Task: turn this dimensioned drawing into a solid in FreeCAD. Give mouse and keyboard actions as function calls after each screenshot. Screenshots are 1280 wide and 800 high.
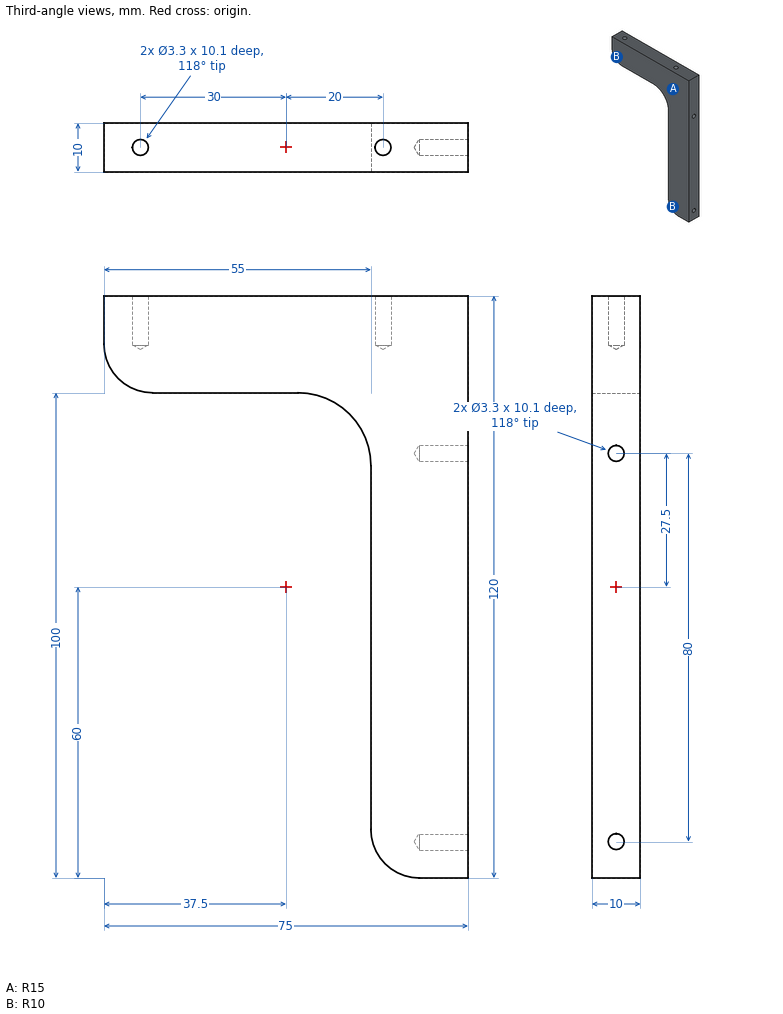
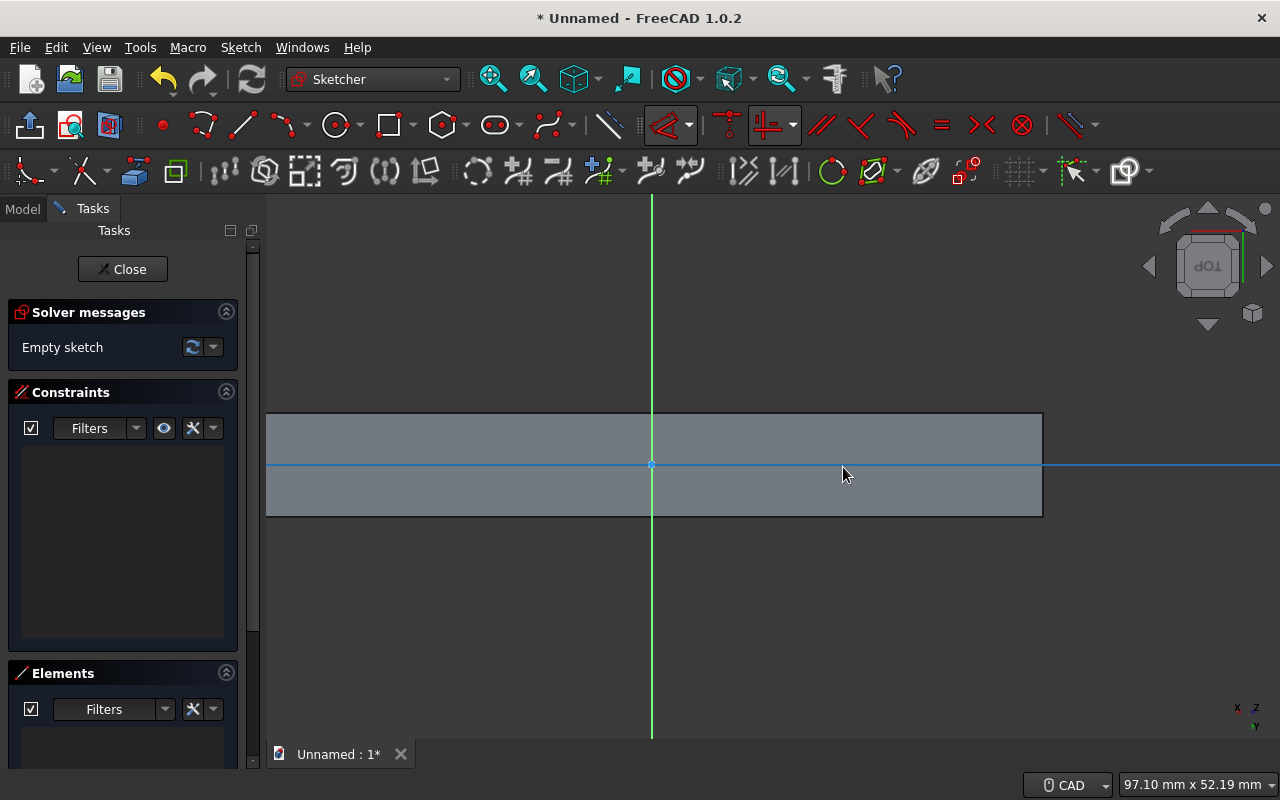
click(336, 126)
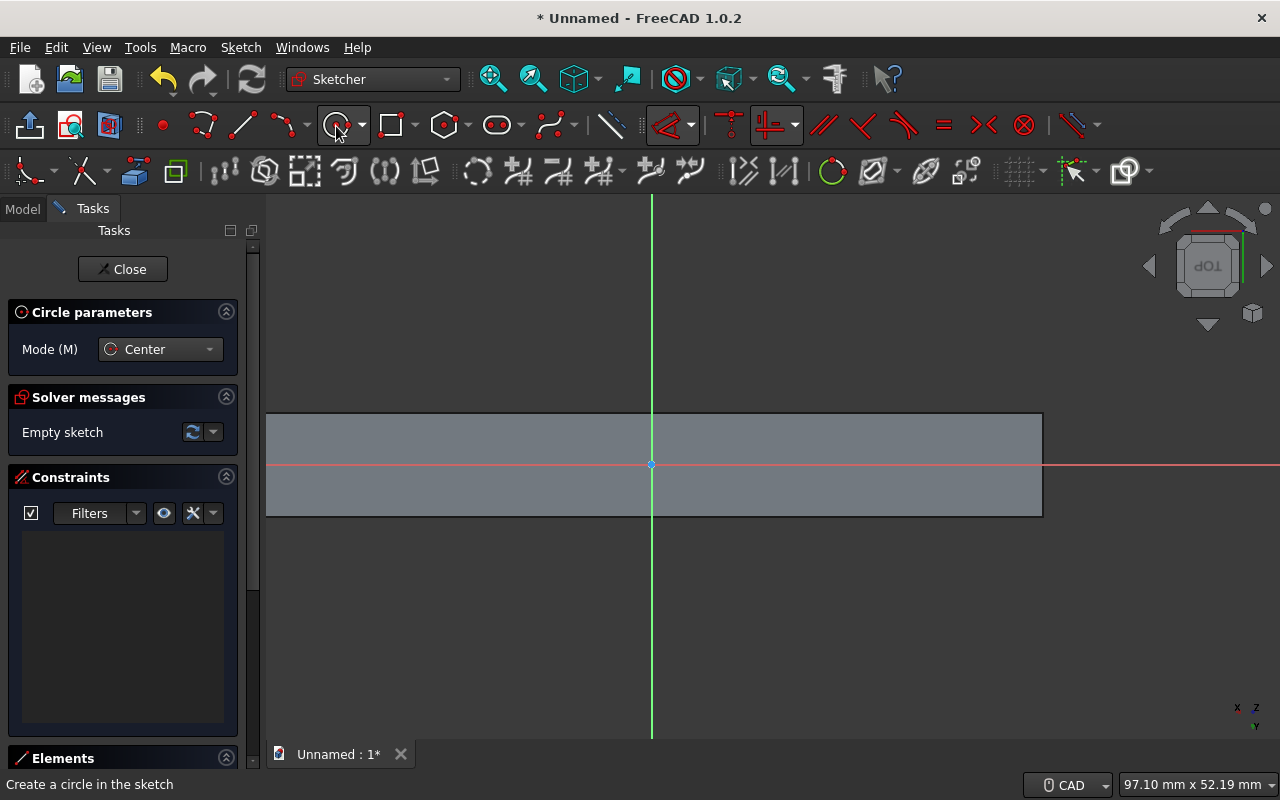
scroll(965, 465, up, 2)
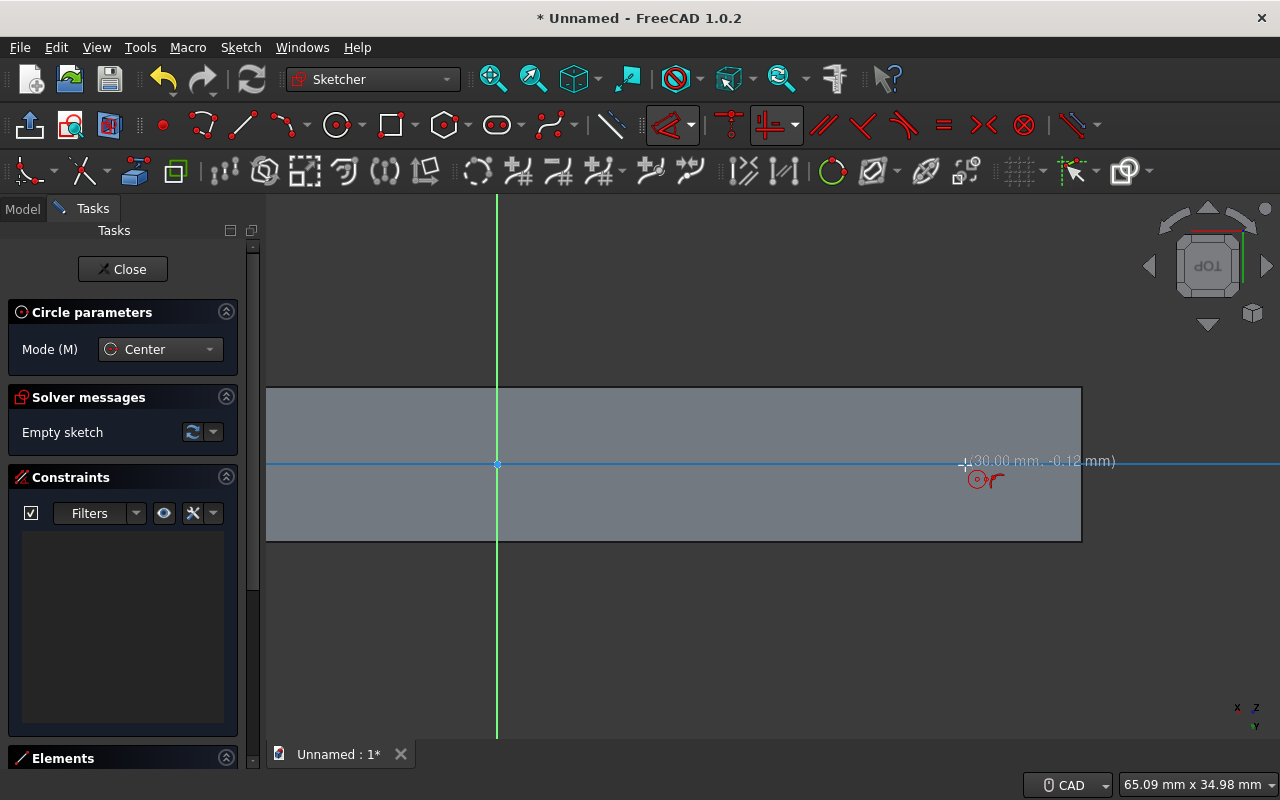
click(965, 464)
click(983, 446)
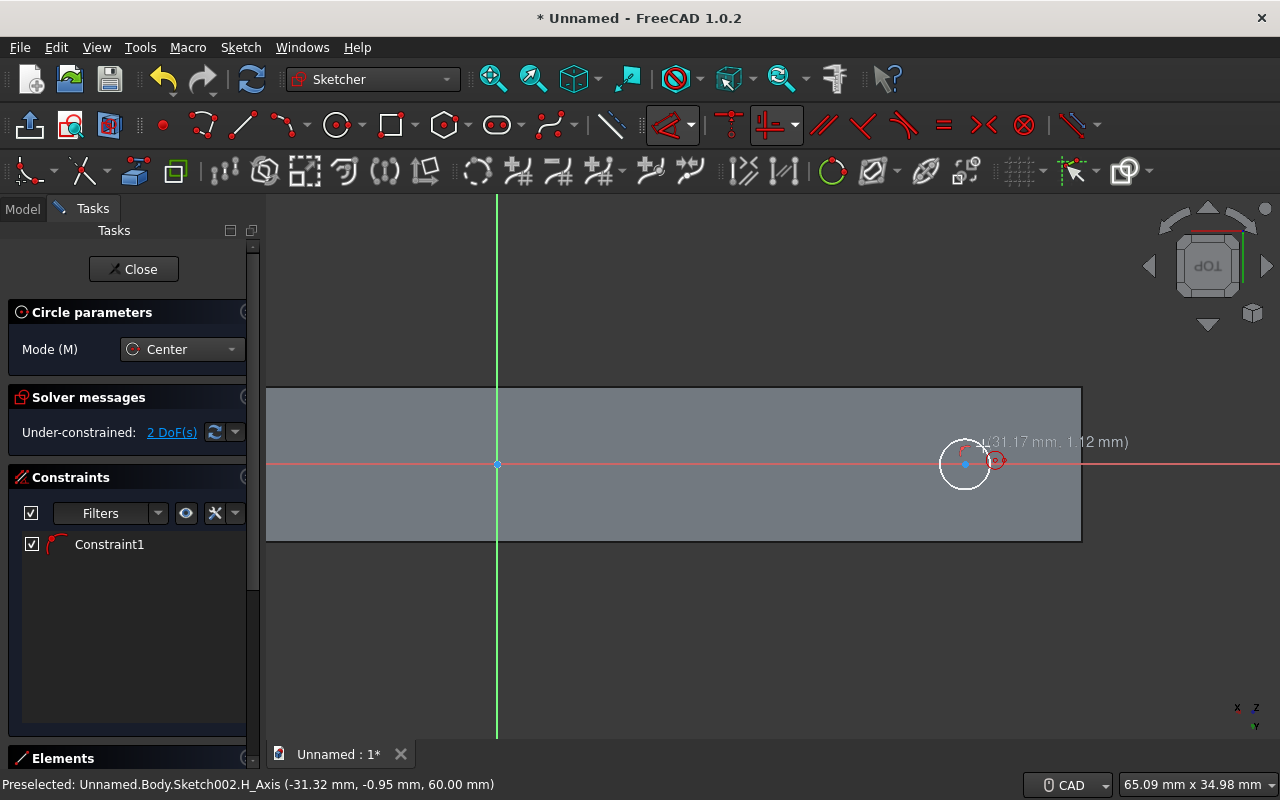
scroll(967, 471, down, 2)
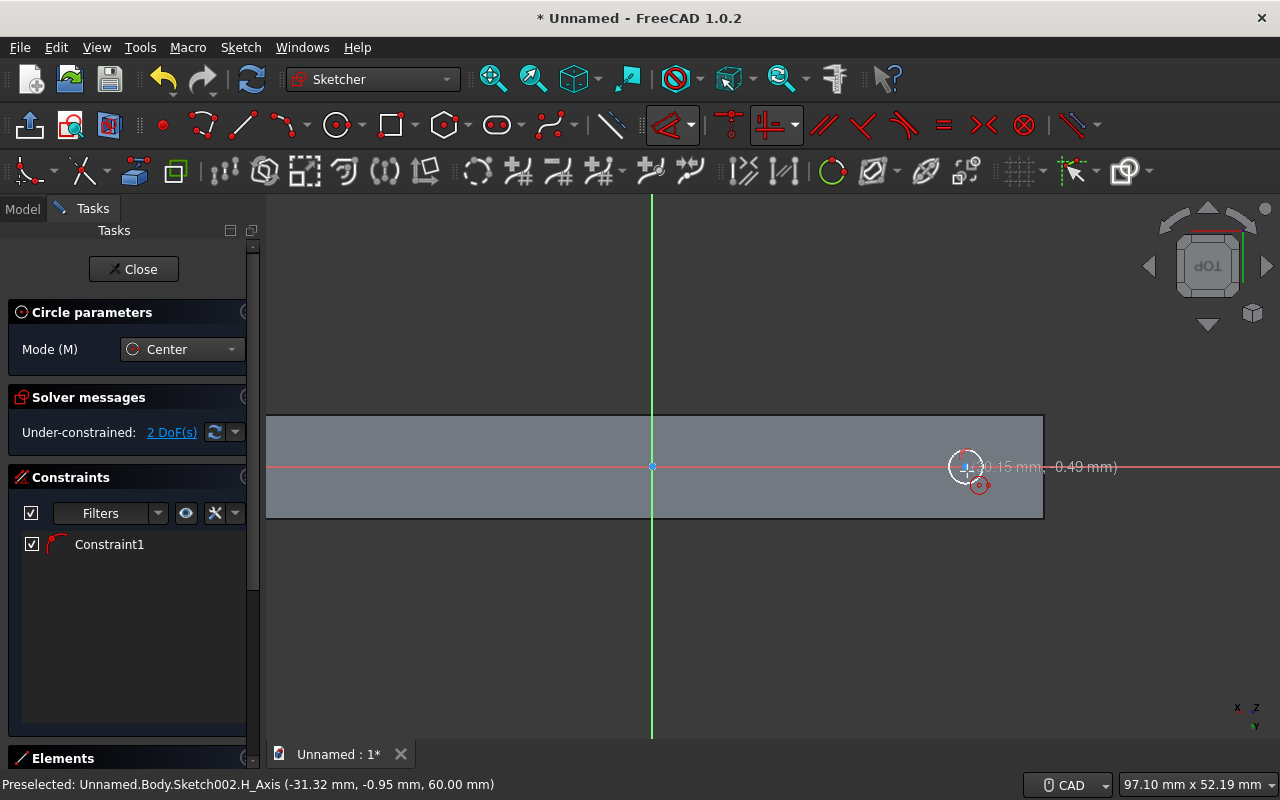
scroll(444, 467, up, 2)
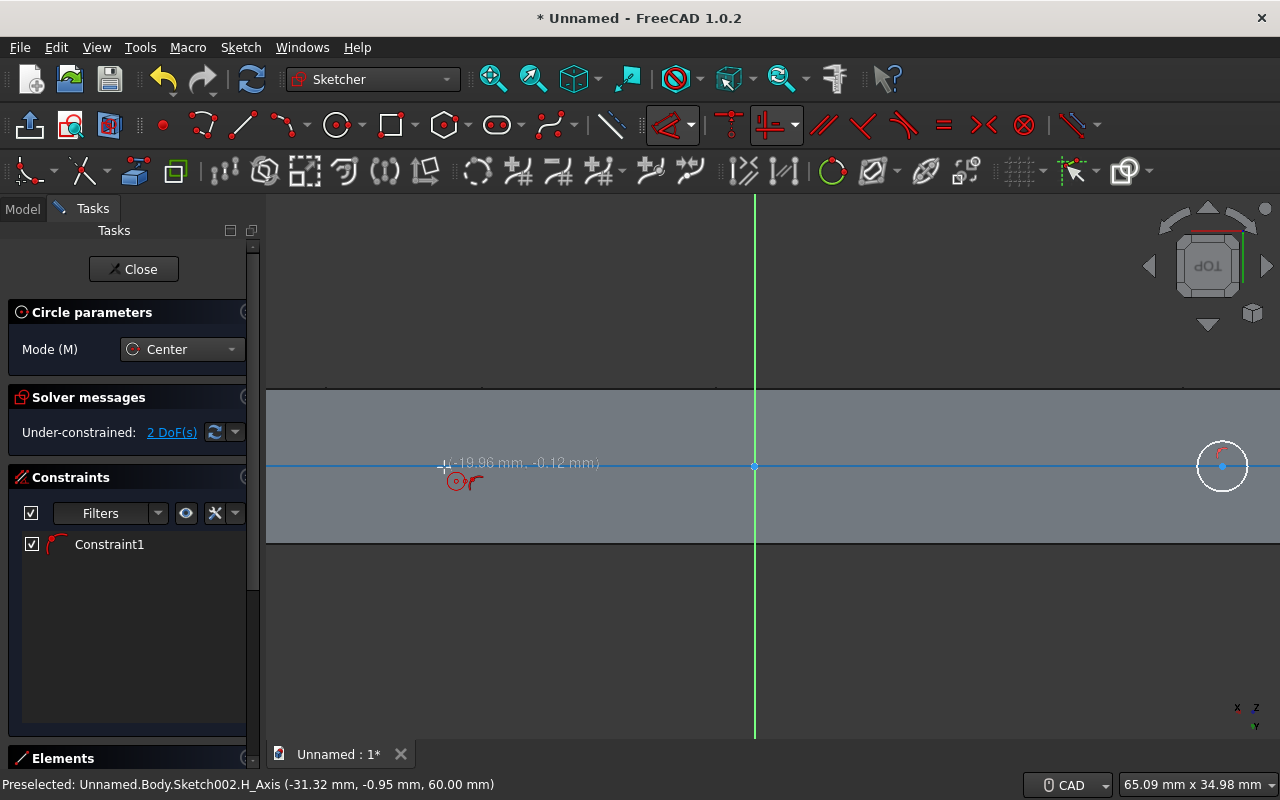
click(443, 466)
click(461, 448)
key(Escape)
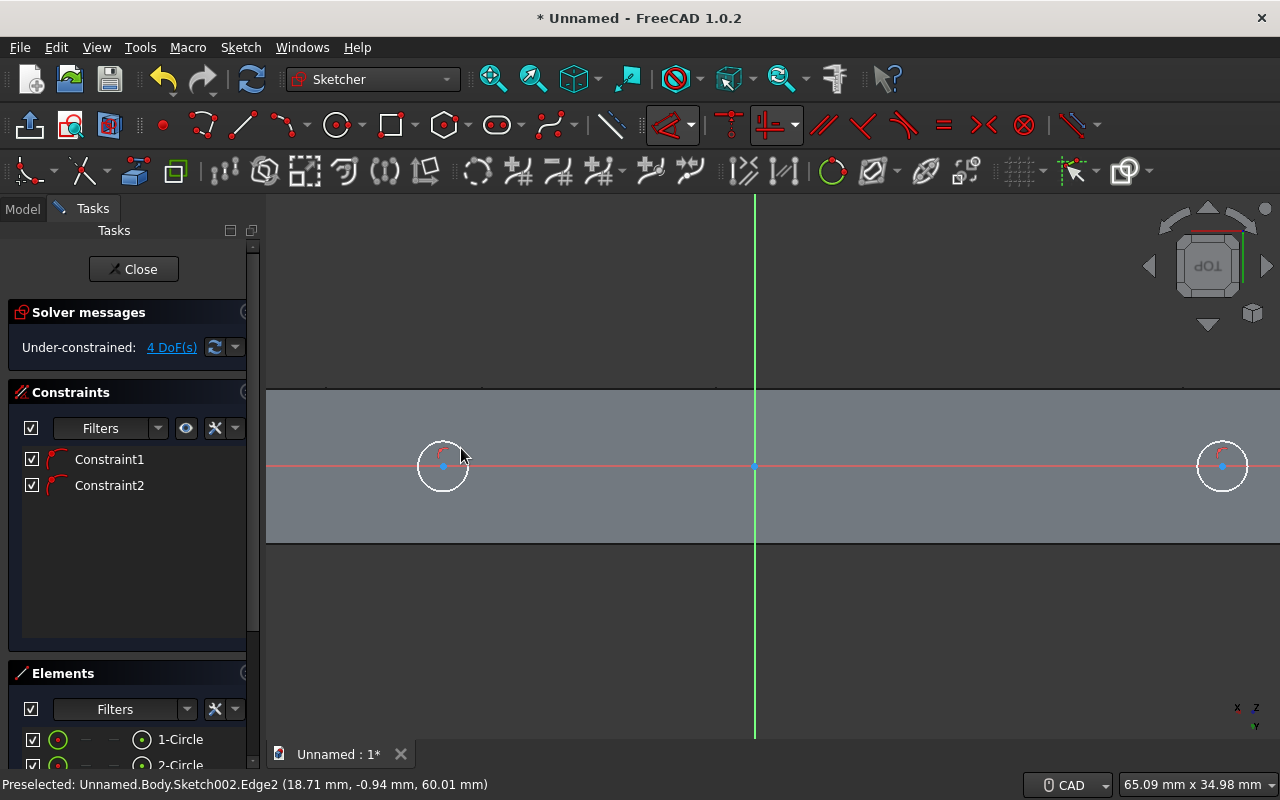
scroll(444, 467, down, 2)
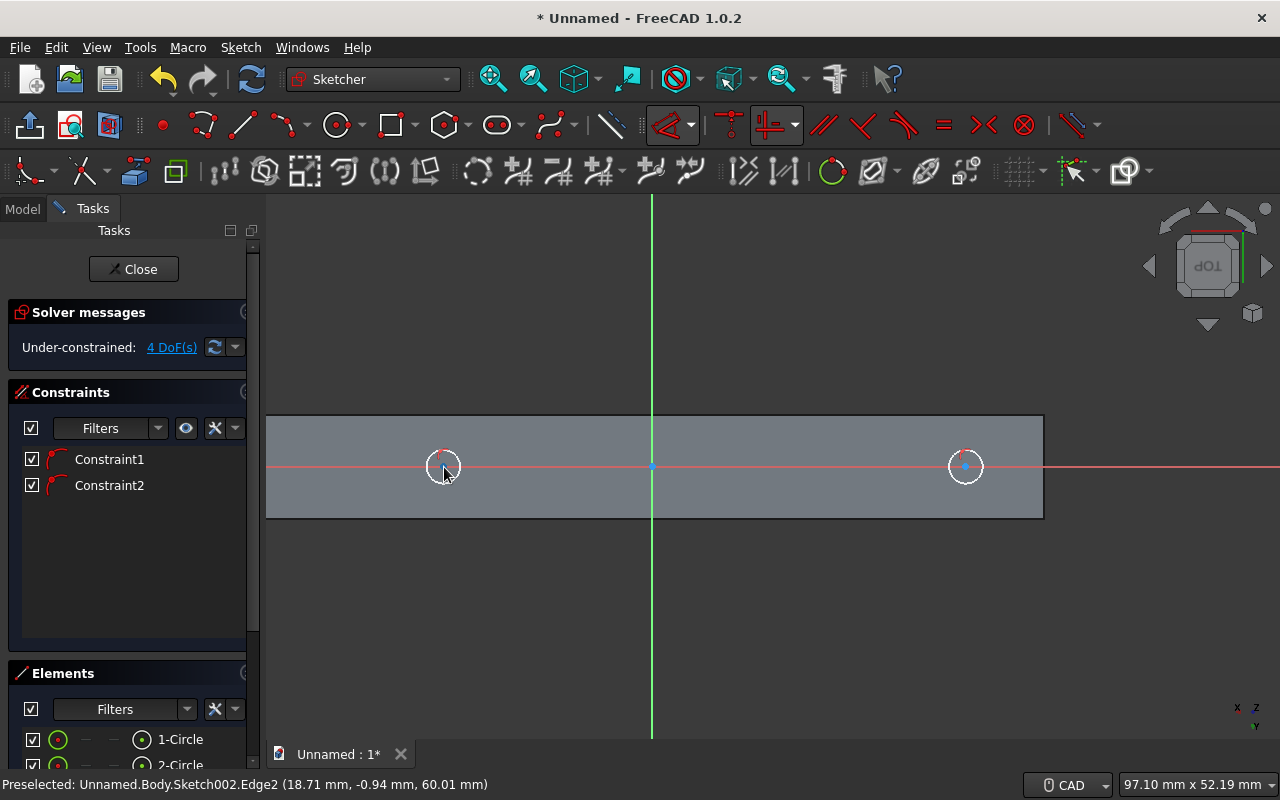
click(978, 455)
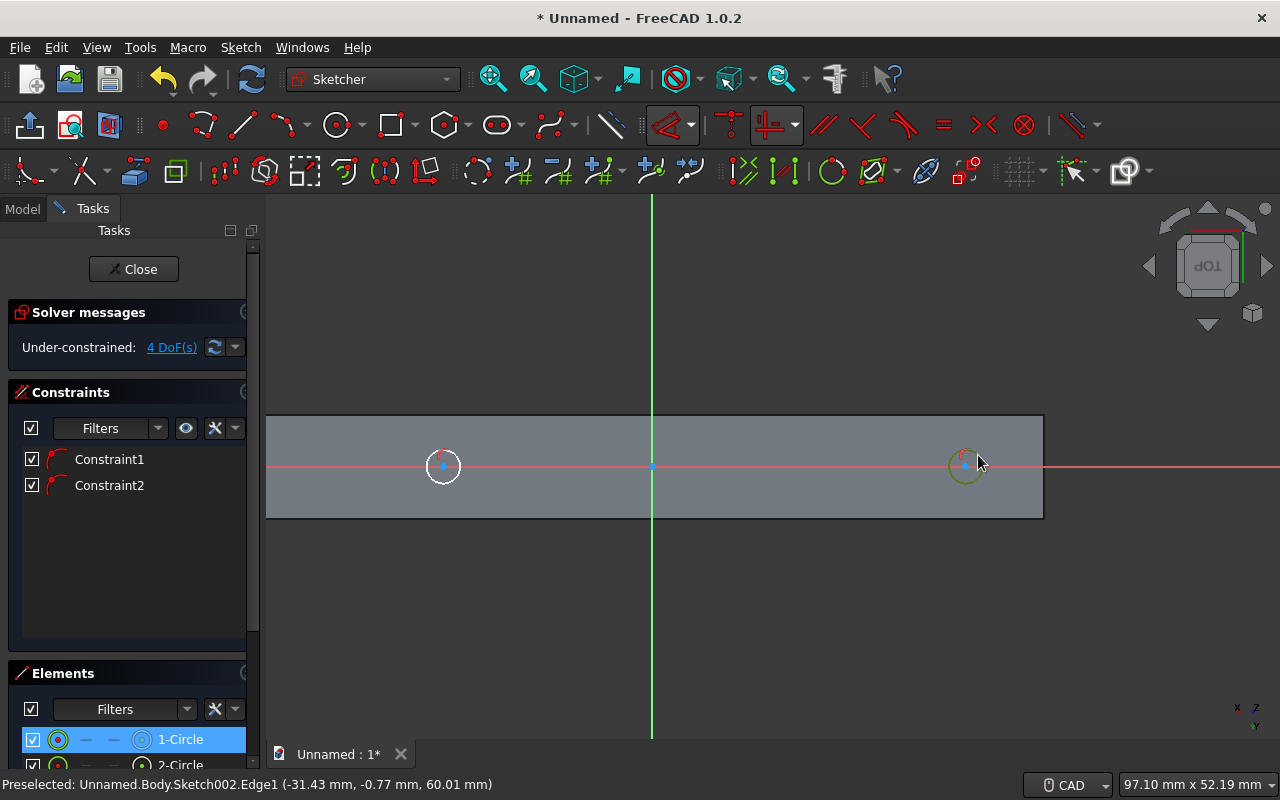
click(455, 455)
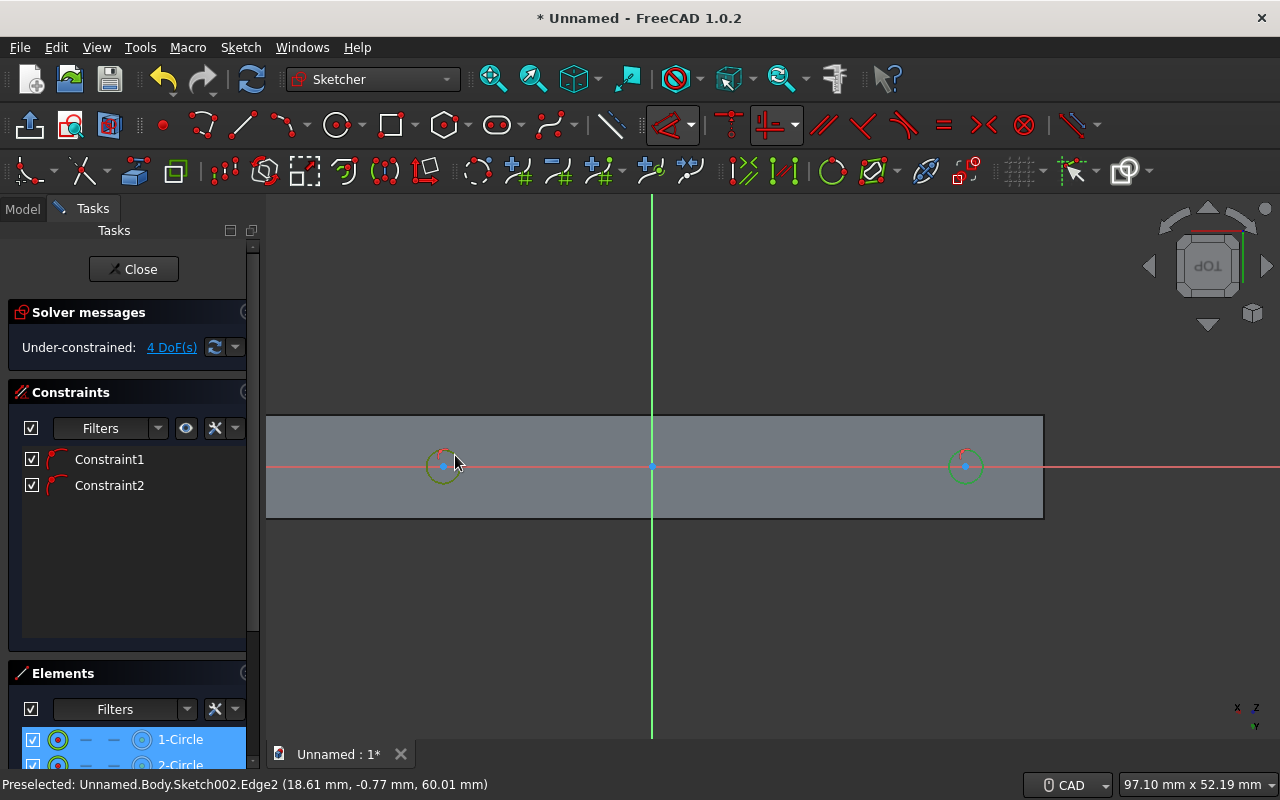
key(e)